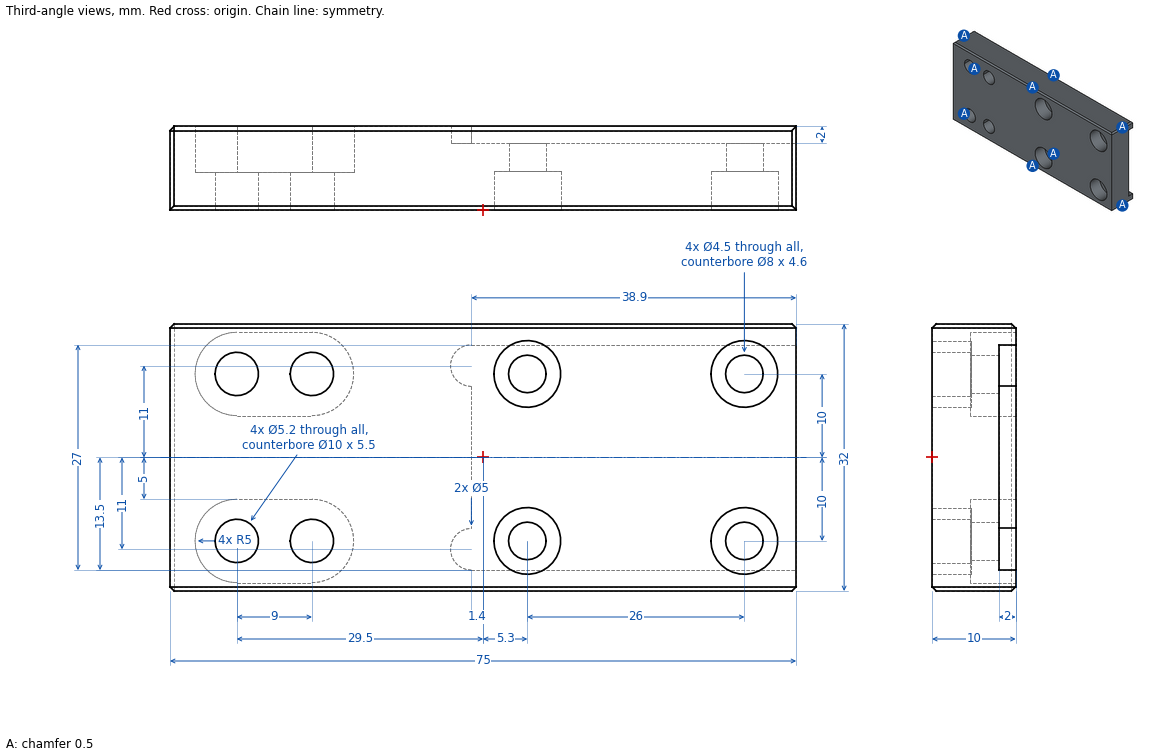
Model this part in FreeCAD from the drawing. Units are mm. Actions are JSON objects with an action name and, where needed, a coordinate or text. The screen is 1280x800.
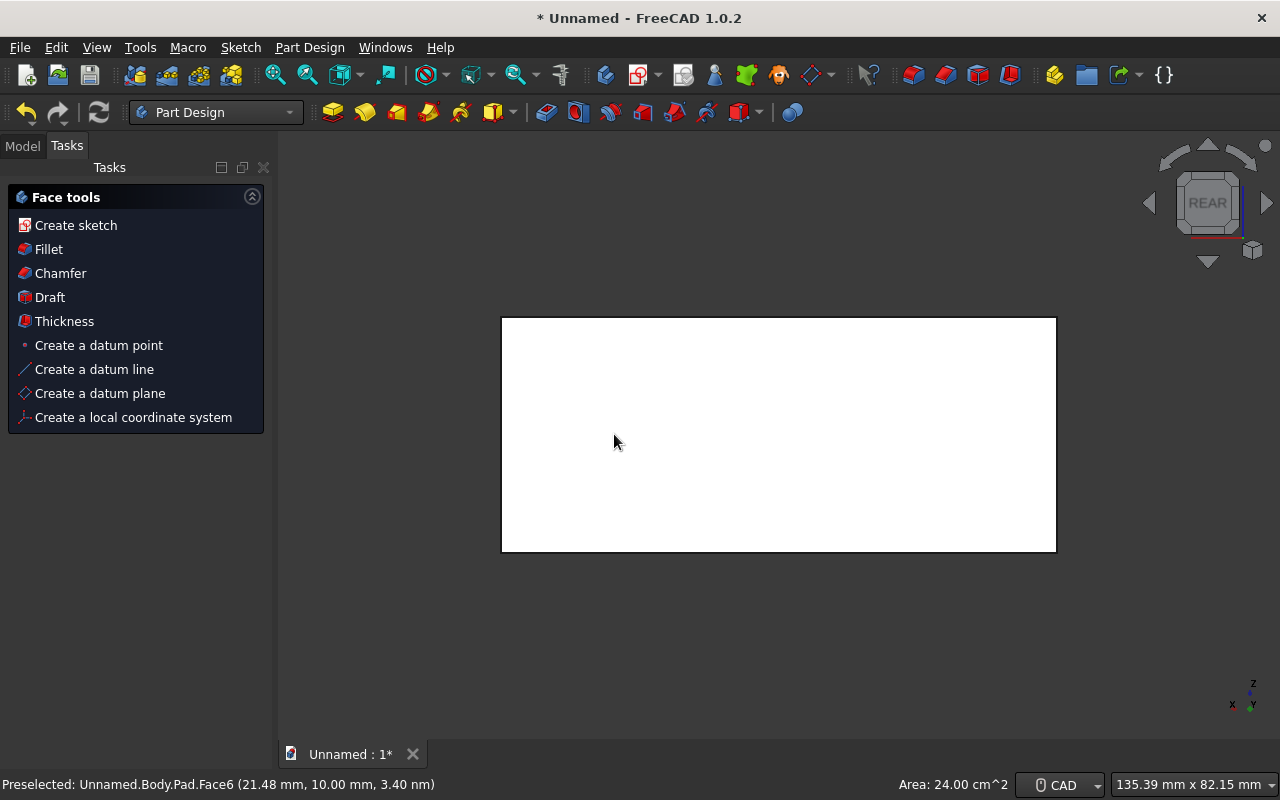
{"action": "left_click", "coordinate": [638, 76]}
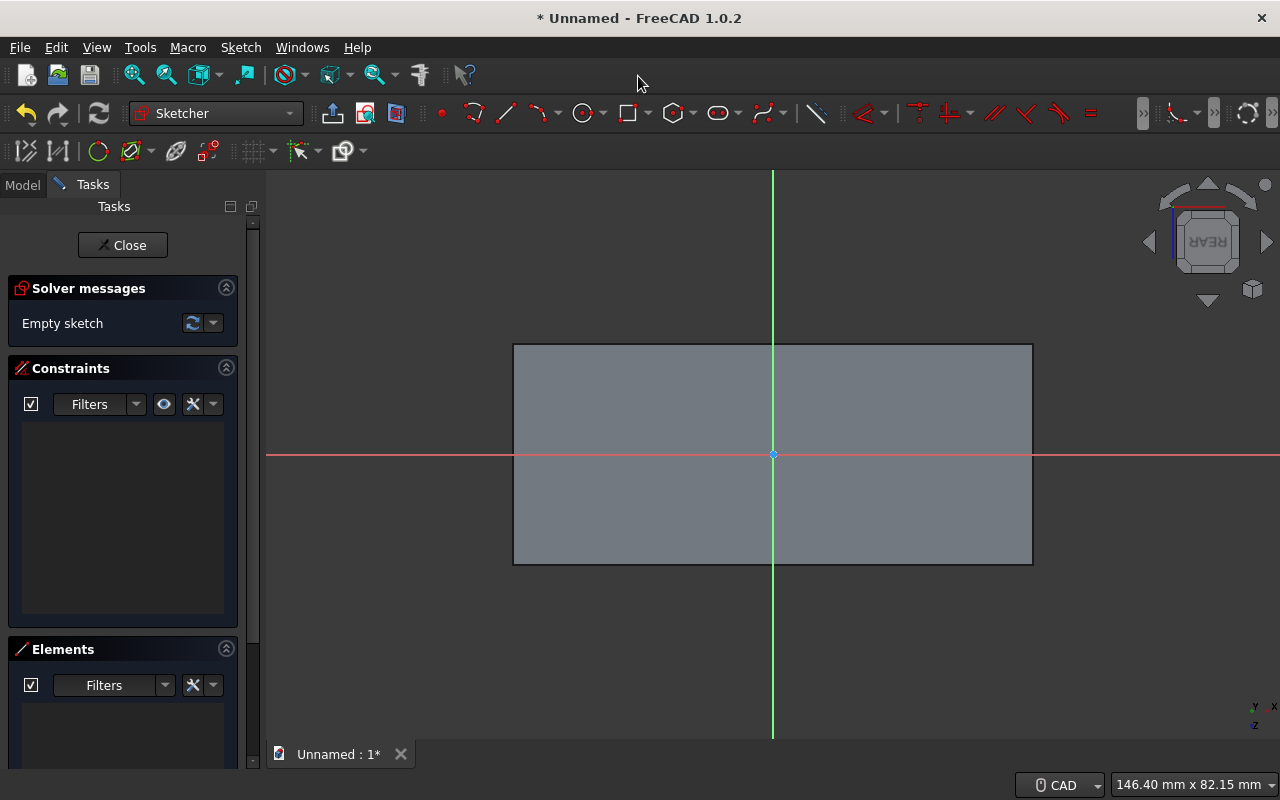
{"action": "scroll", "coordinate": [1115, 454], "scroll_direction": "up", "scroll_amount": 3}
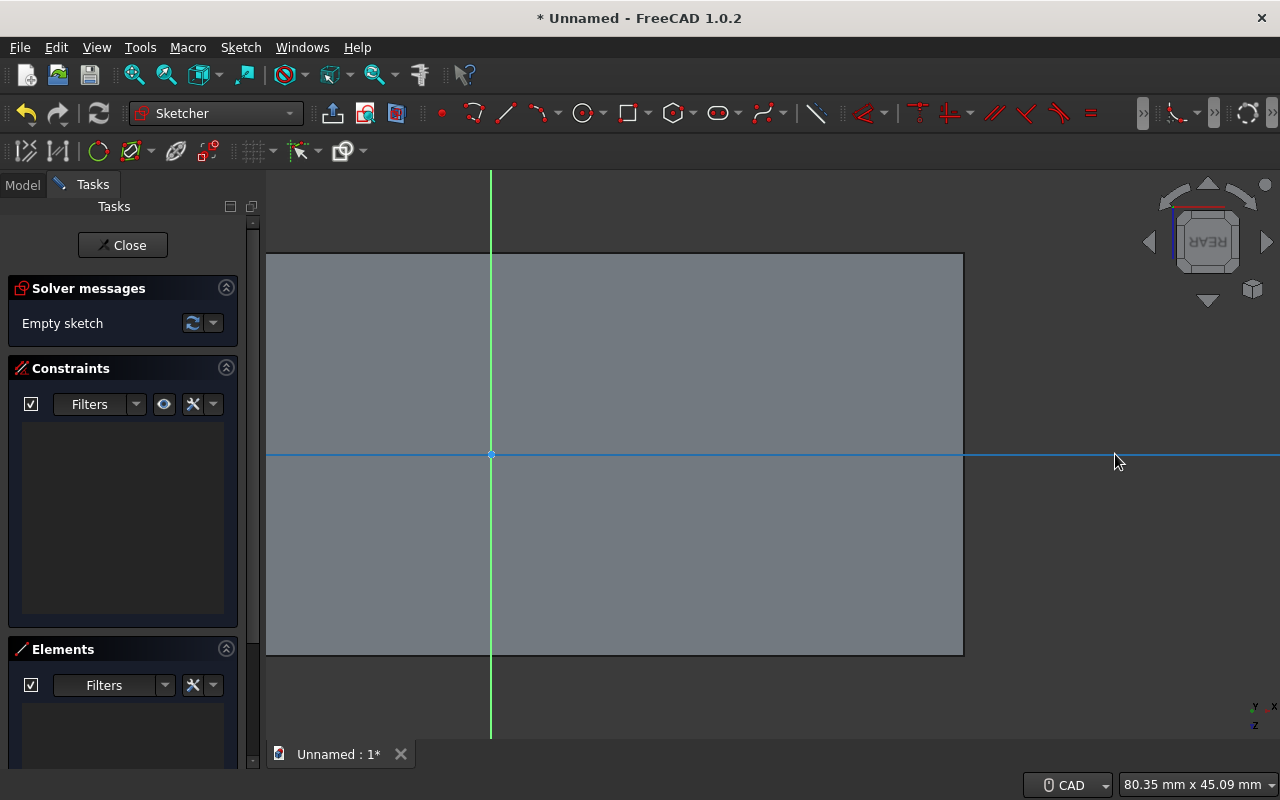
{"action": "left_click", "coordinate": [628, 114]}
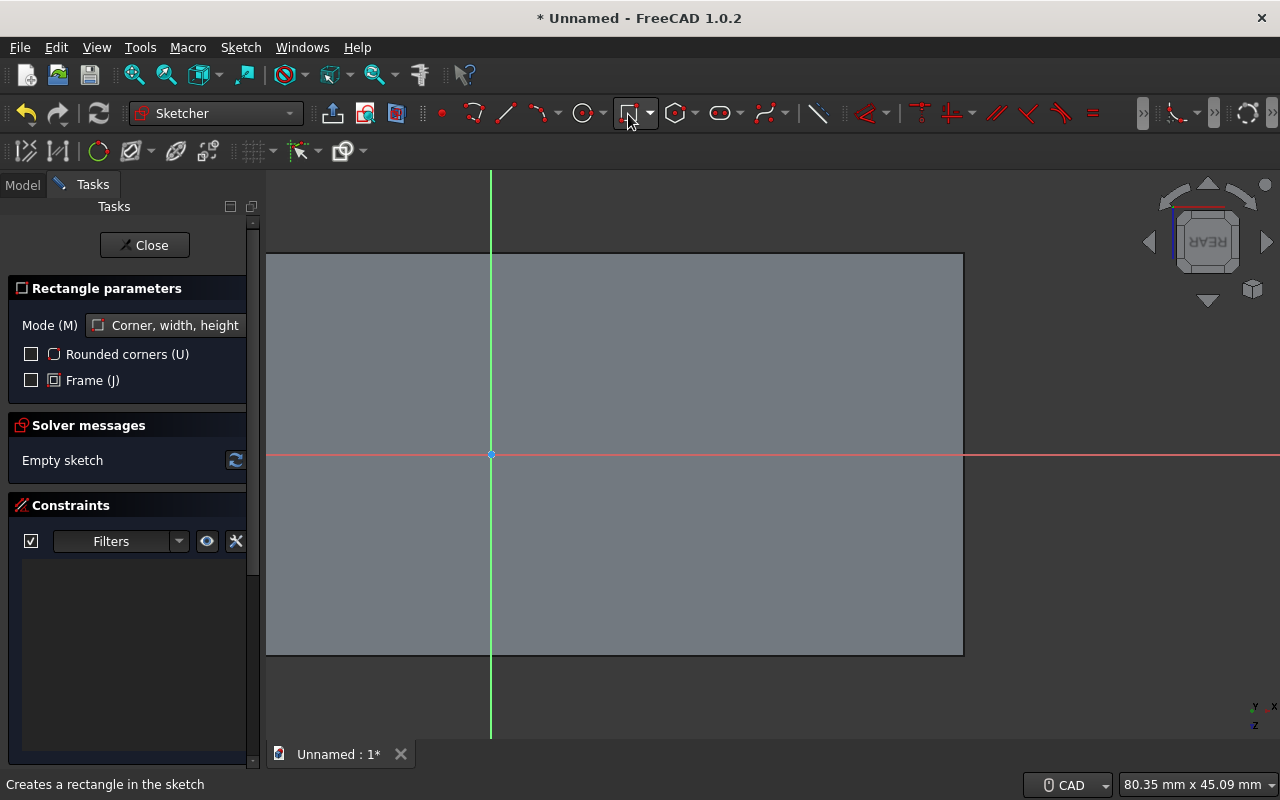
{"action": "left_click", "coordinate": [473, 284]}
{"action": "left_click", "coordinate": [964, 625]}
{"action": "key", "text": "Escape"}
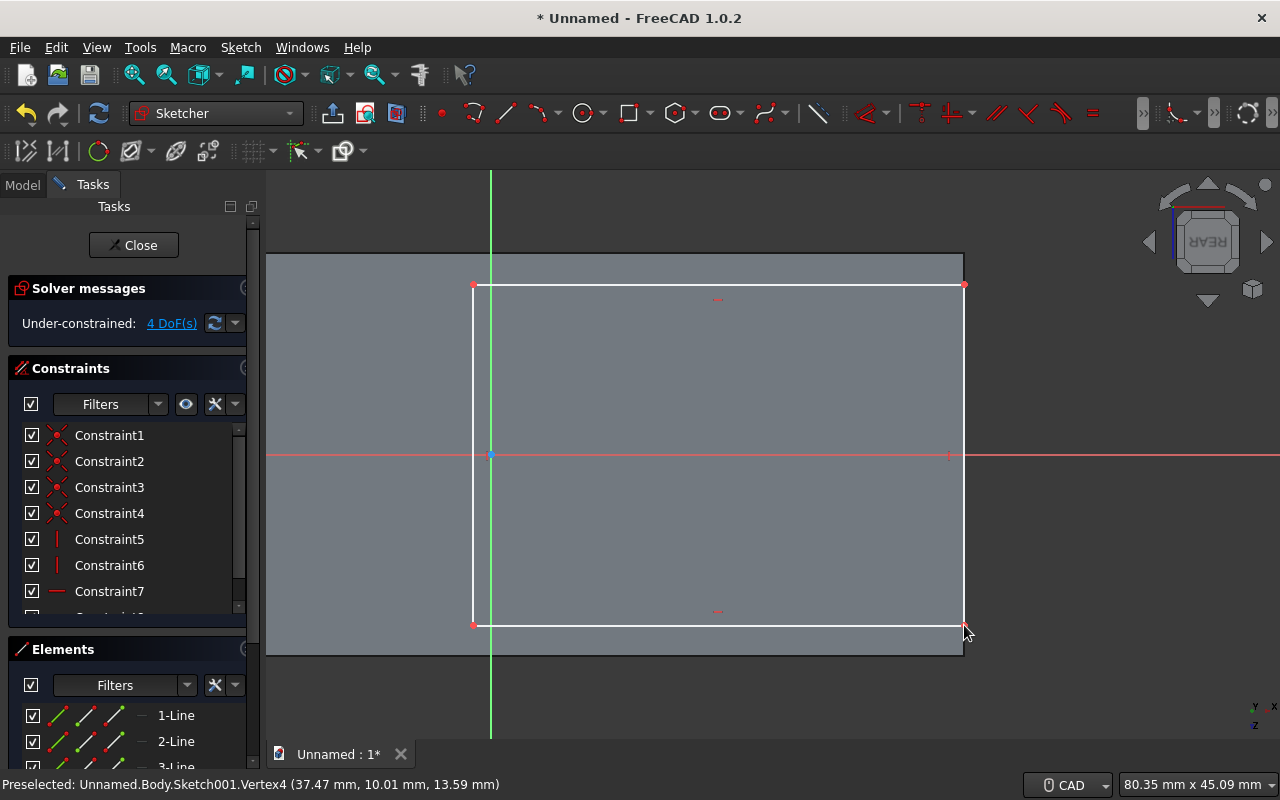
{"action": "left_click", "coordinate": [866, 114]}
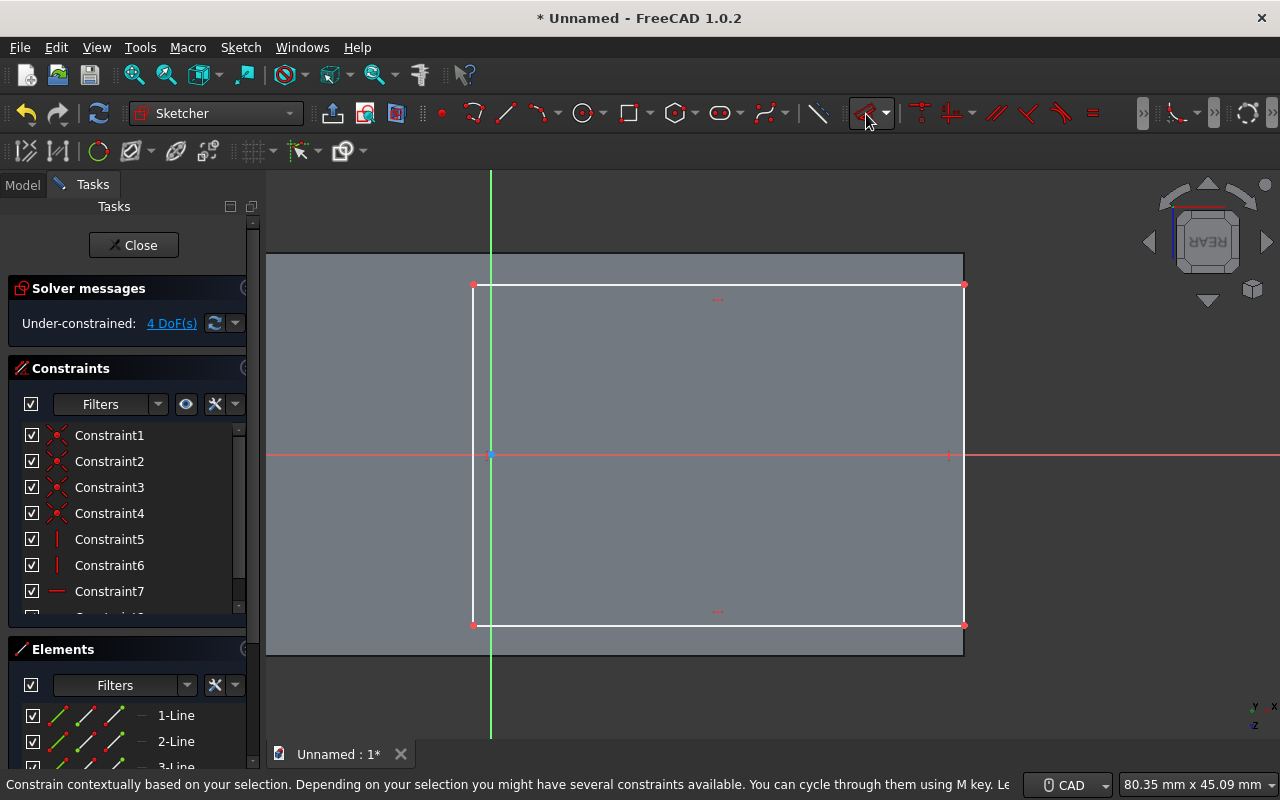
{"action": "left_click", "coordinate": [473, 387]}
{"action": "left_click", "coordinate": [439, 377]}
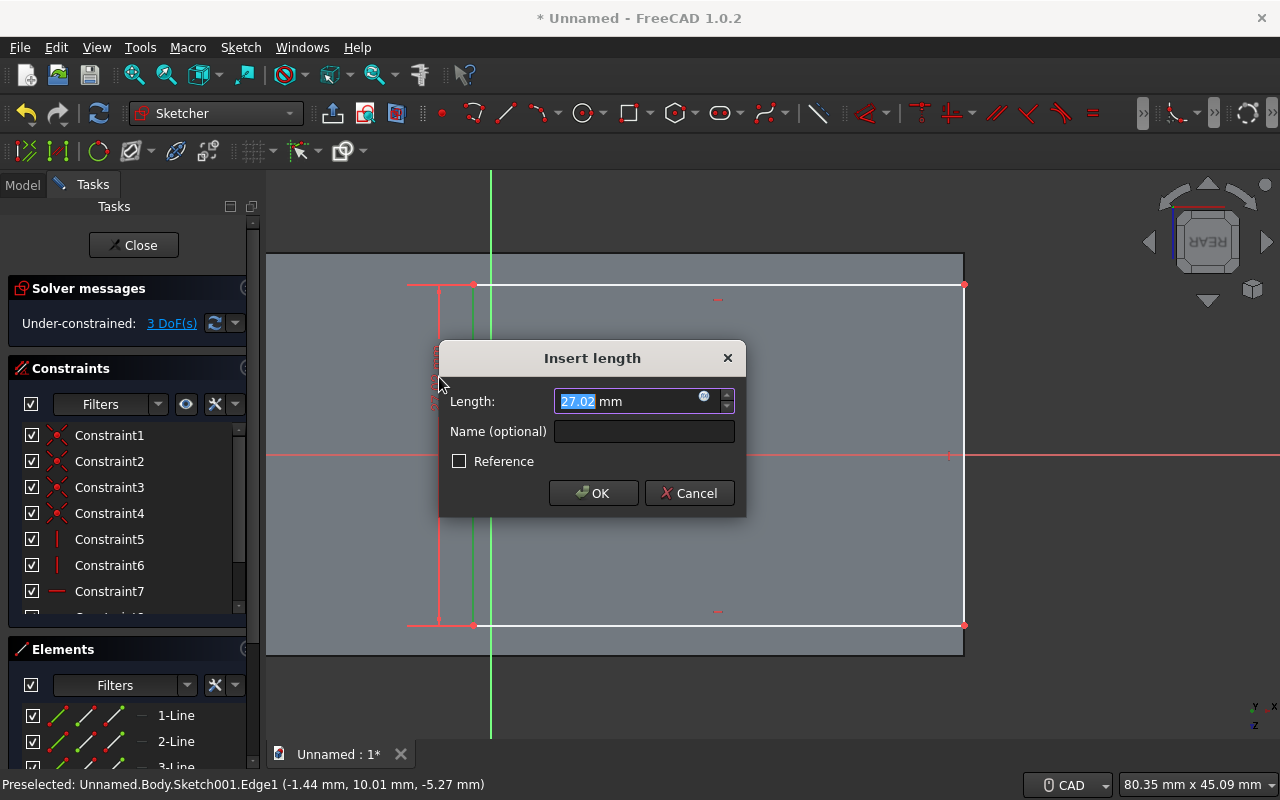
{"action": "type", "text": "27"}
{"action": "key", "text": "Return"}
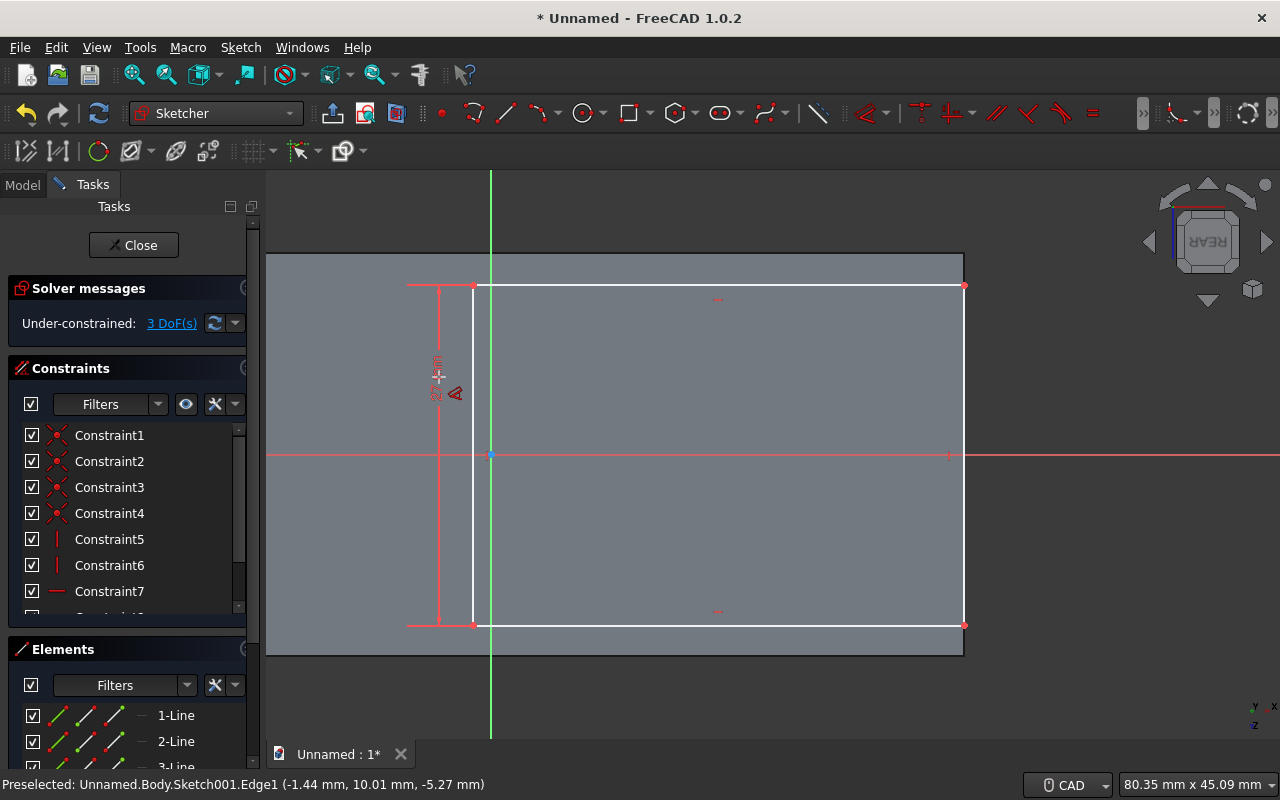
{"action": "left_click", "coordinate": [620, 626]}
{"action": "left_click", "coordinate": [718, 660]}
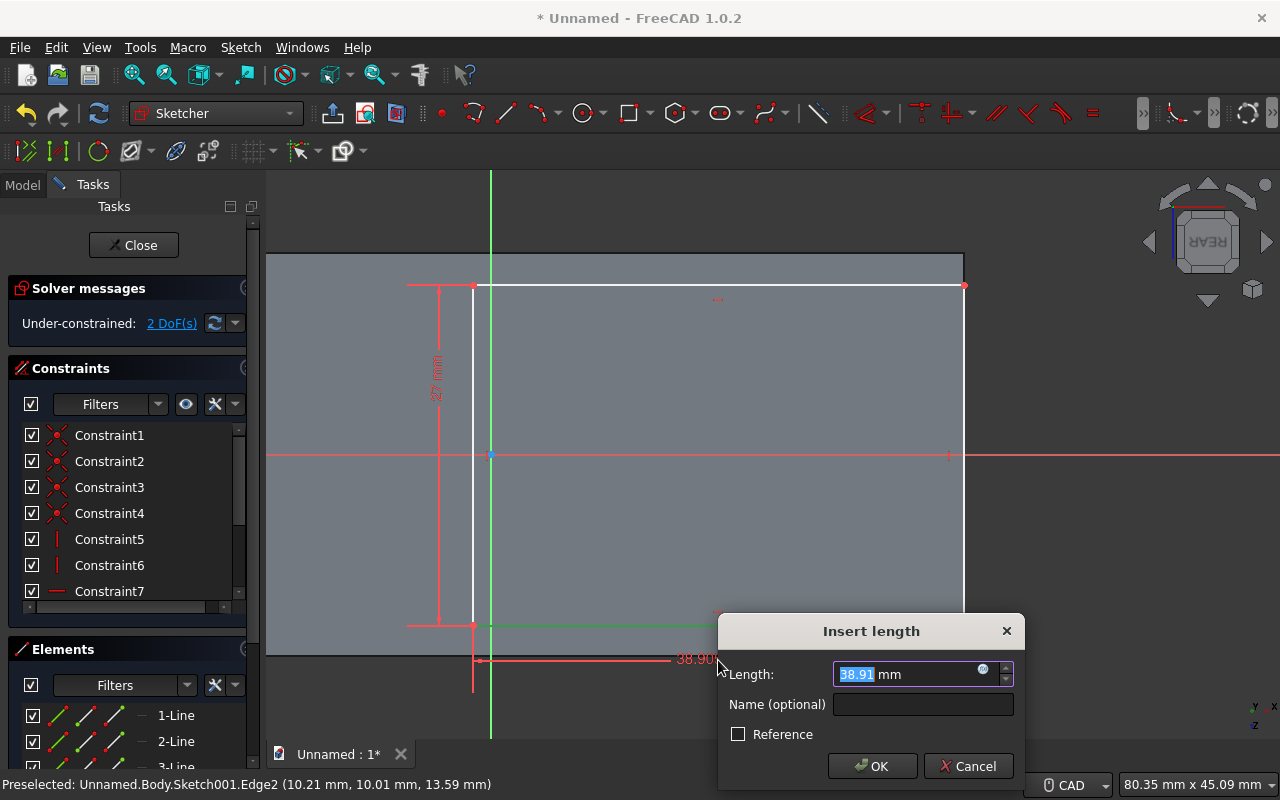
{"action": "type", "text": "38.9"}
{"action": "key", "text": "Return"}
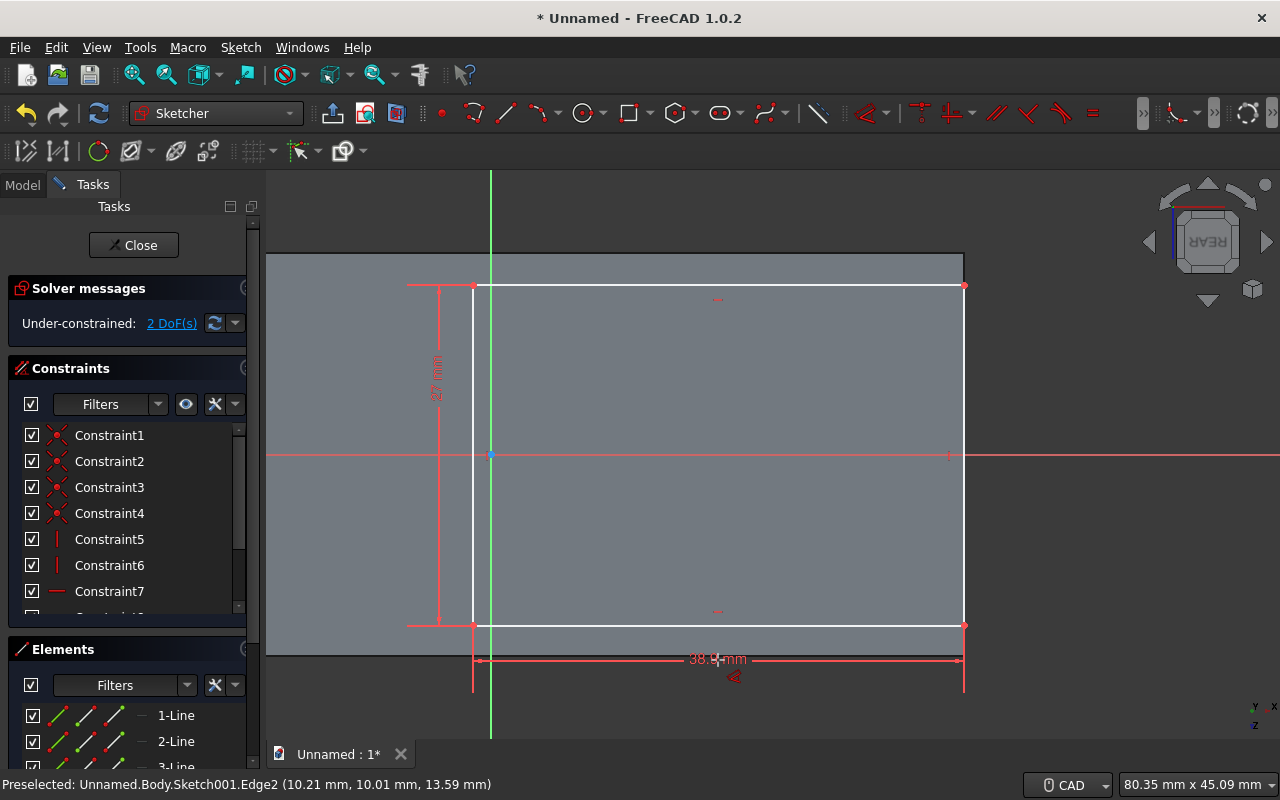
{"action": "scroll", "coordinate": [473, 285], "scroll_direction": "up", "scroll_amount": 5}